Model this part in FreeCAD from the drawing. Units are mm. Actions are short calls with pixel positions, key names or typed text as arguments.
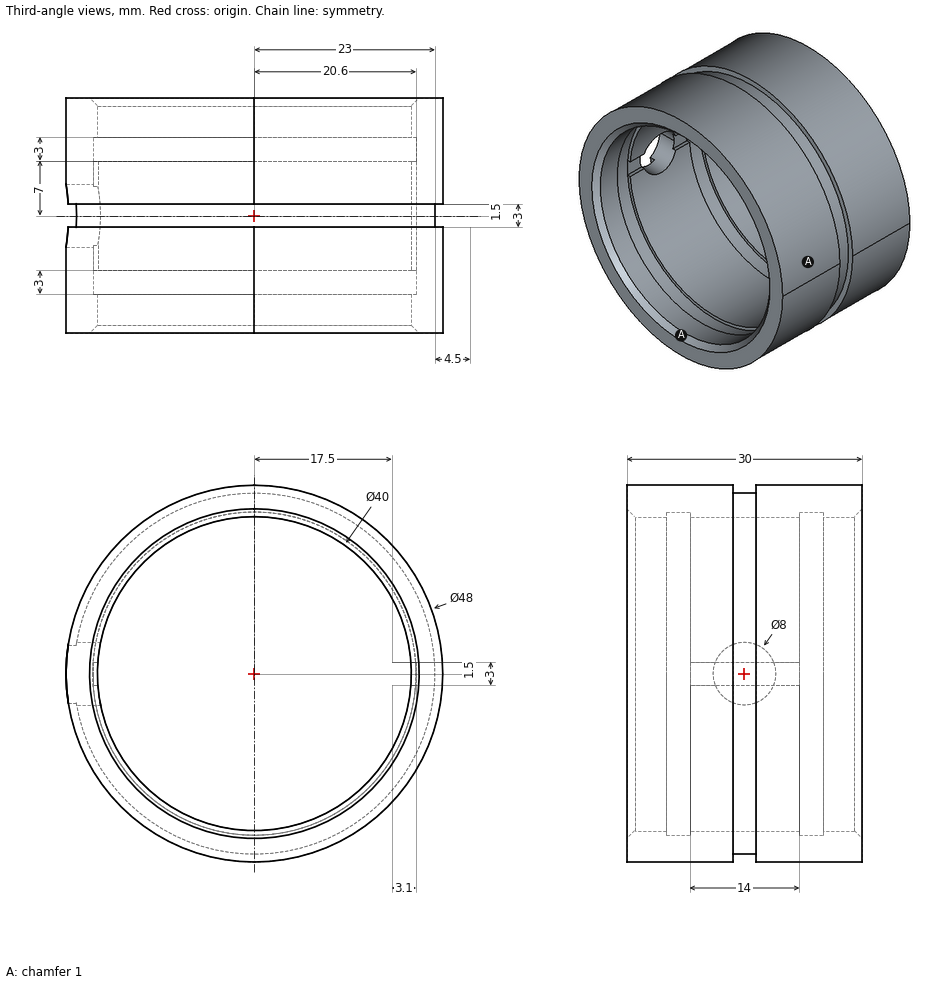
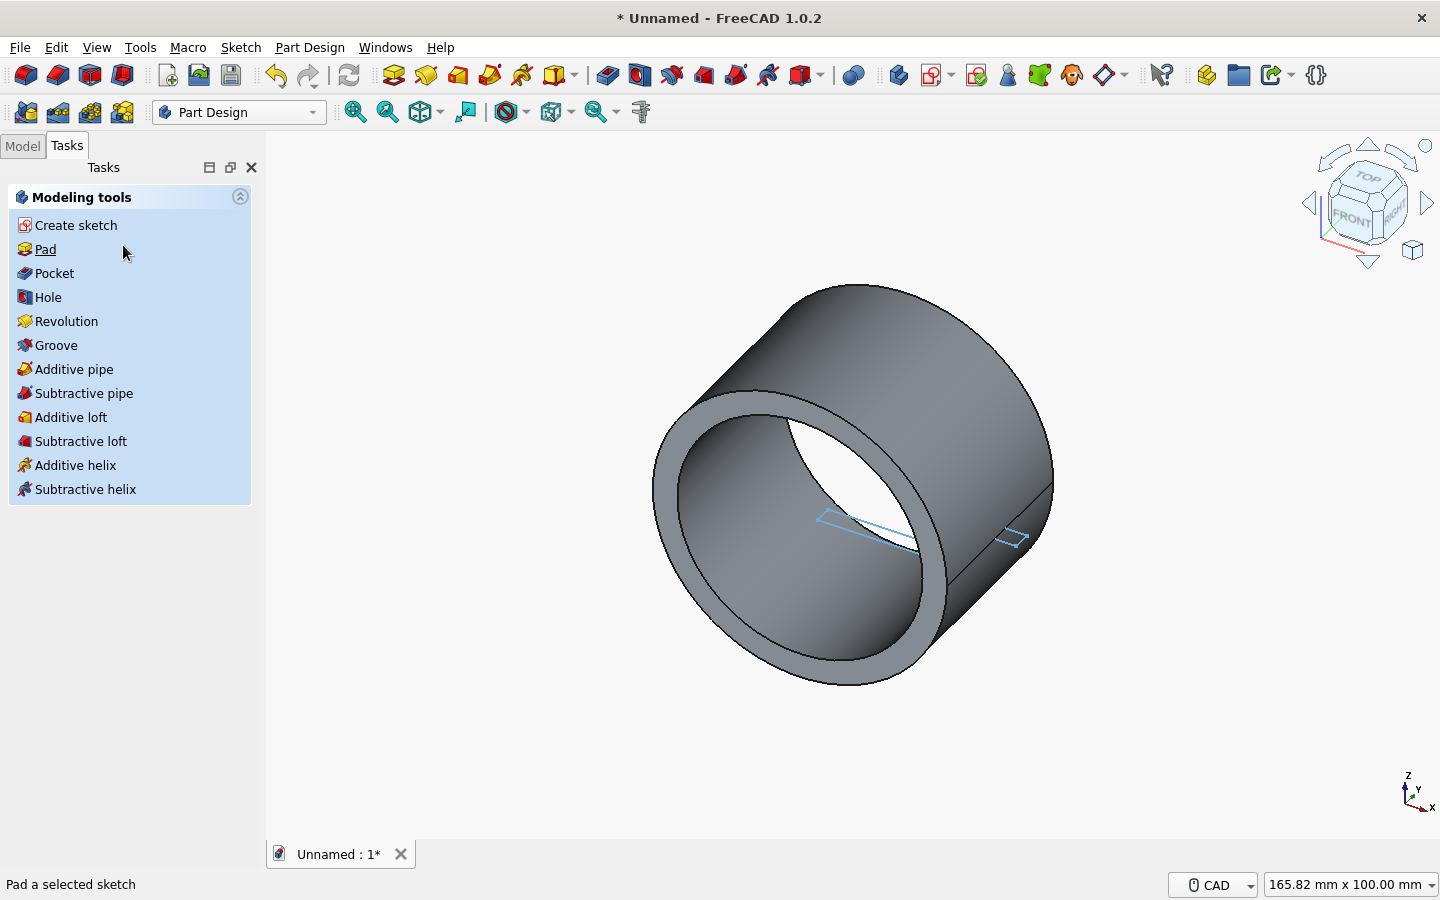
click(672, 76)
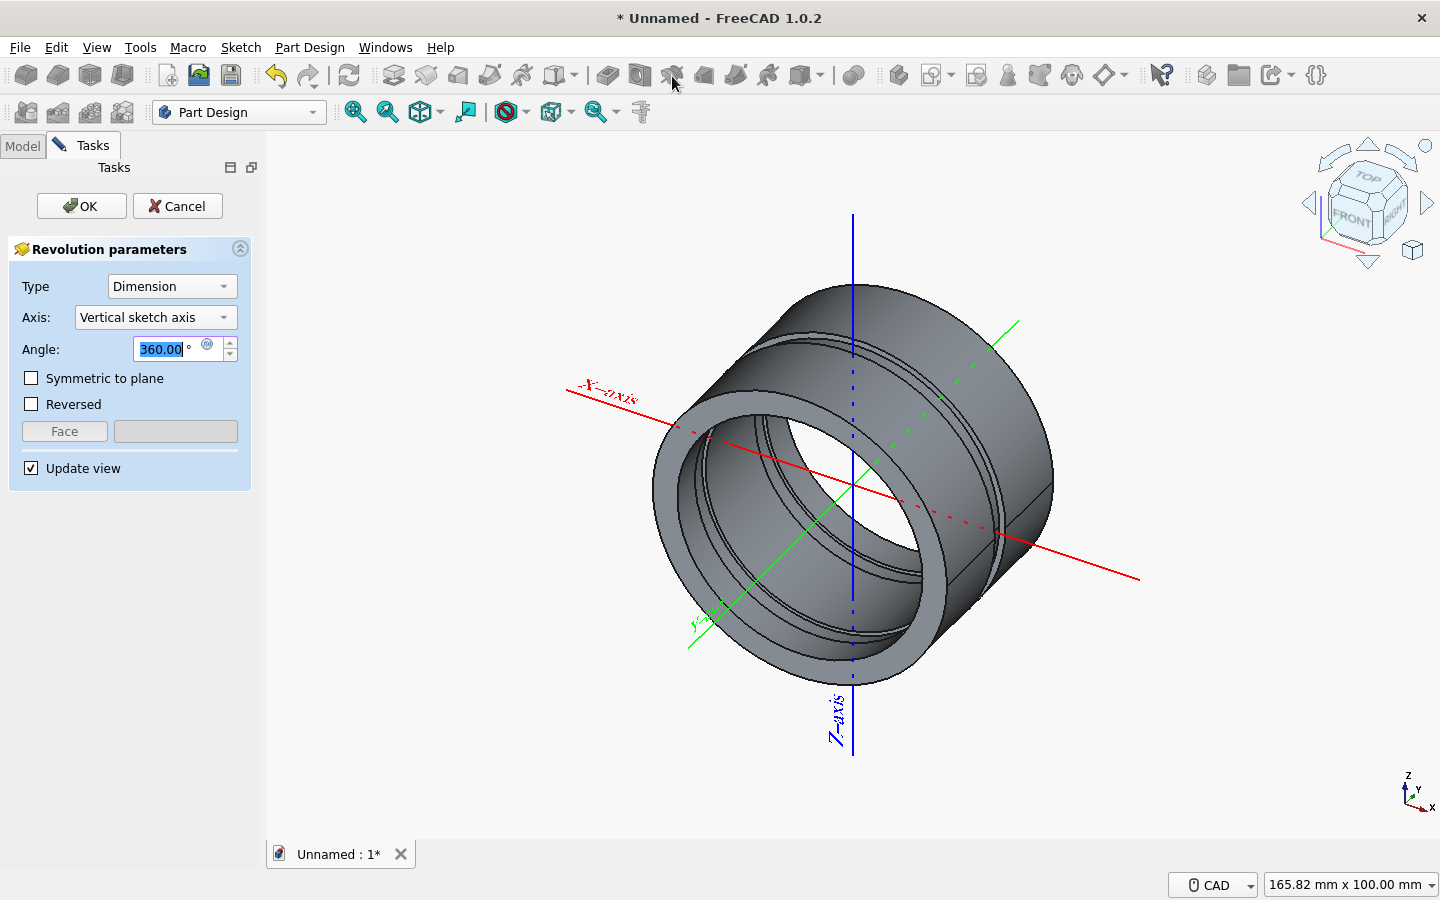
click(82, 206)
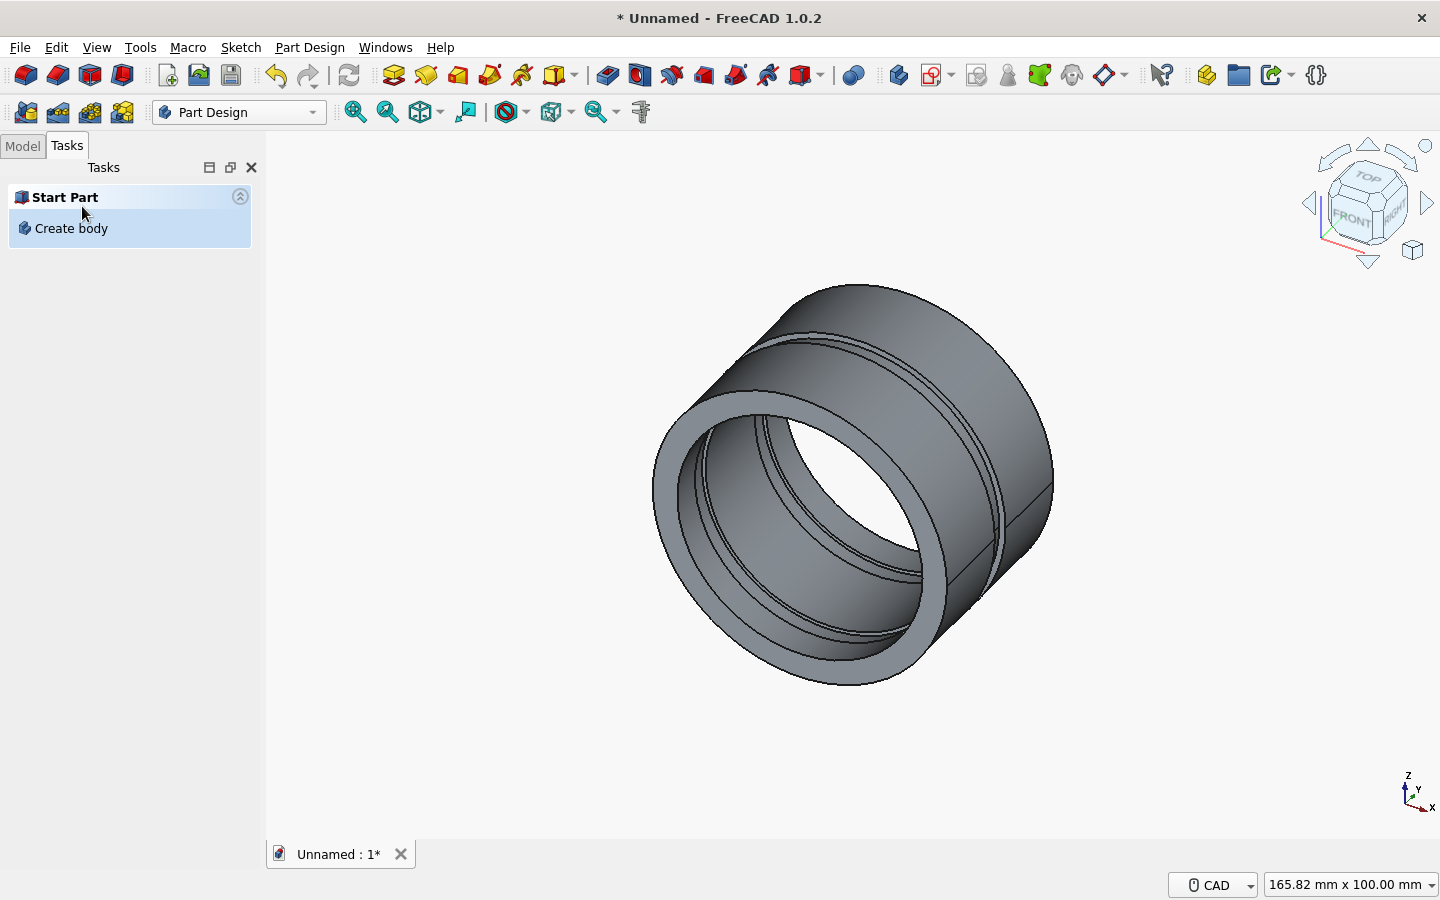
click(932, 76)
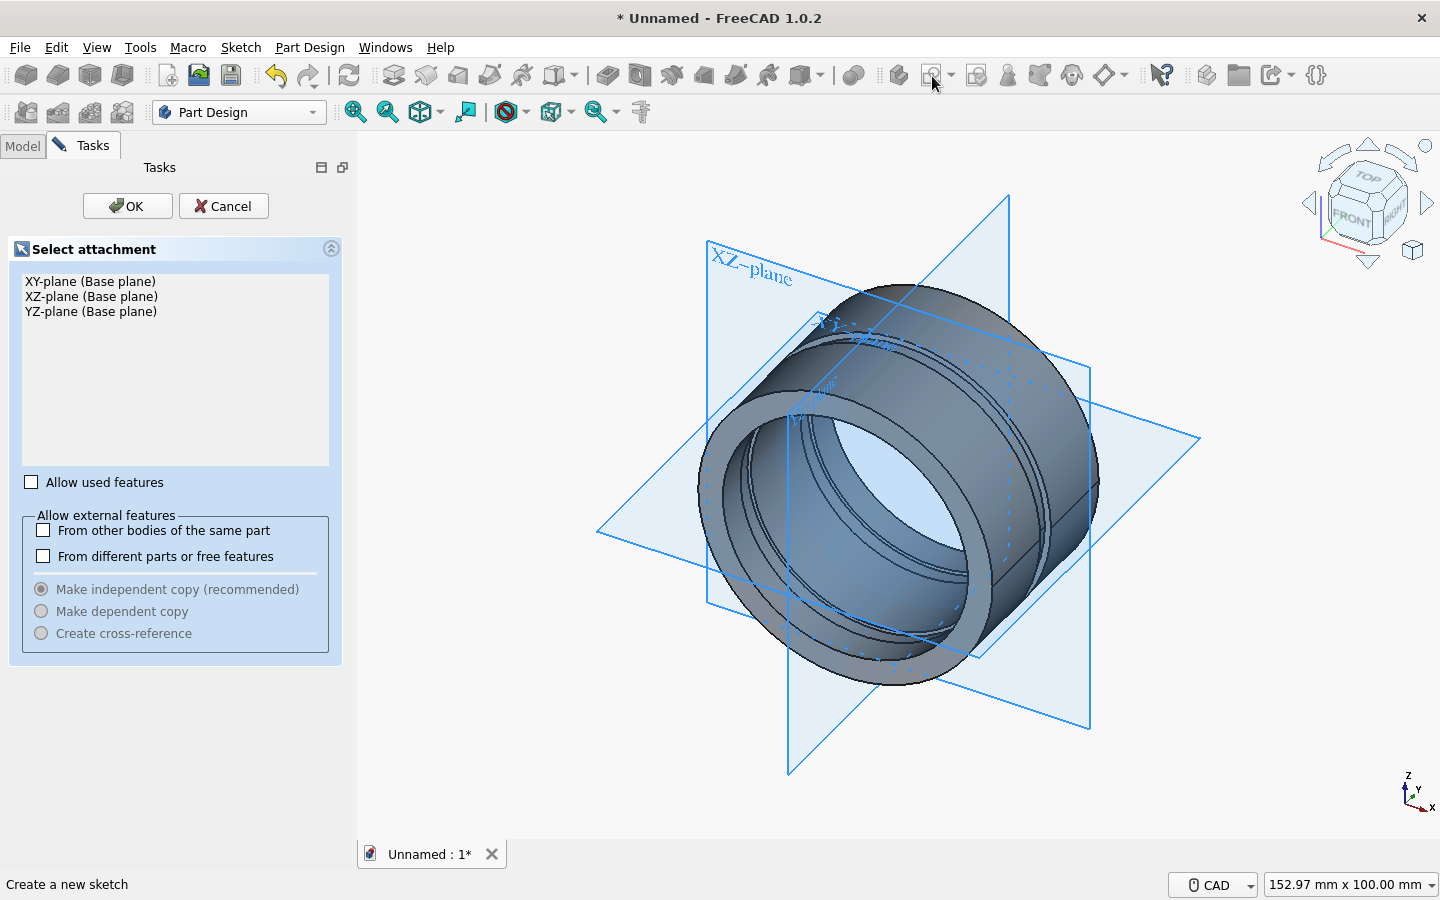
click(82, 296)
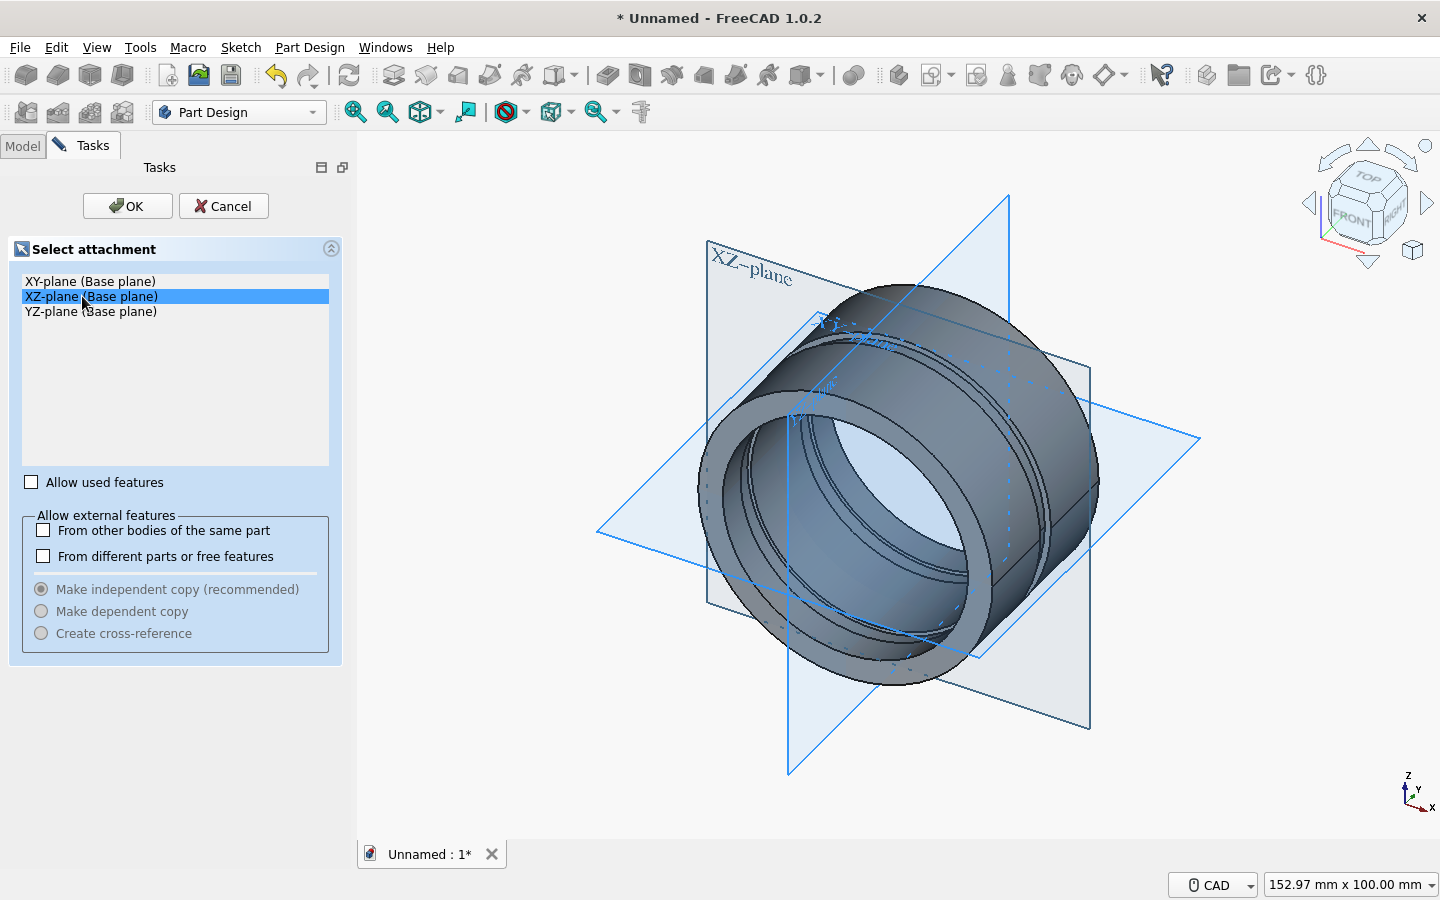
click(128, 206)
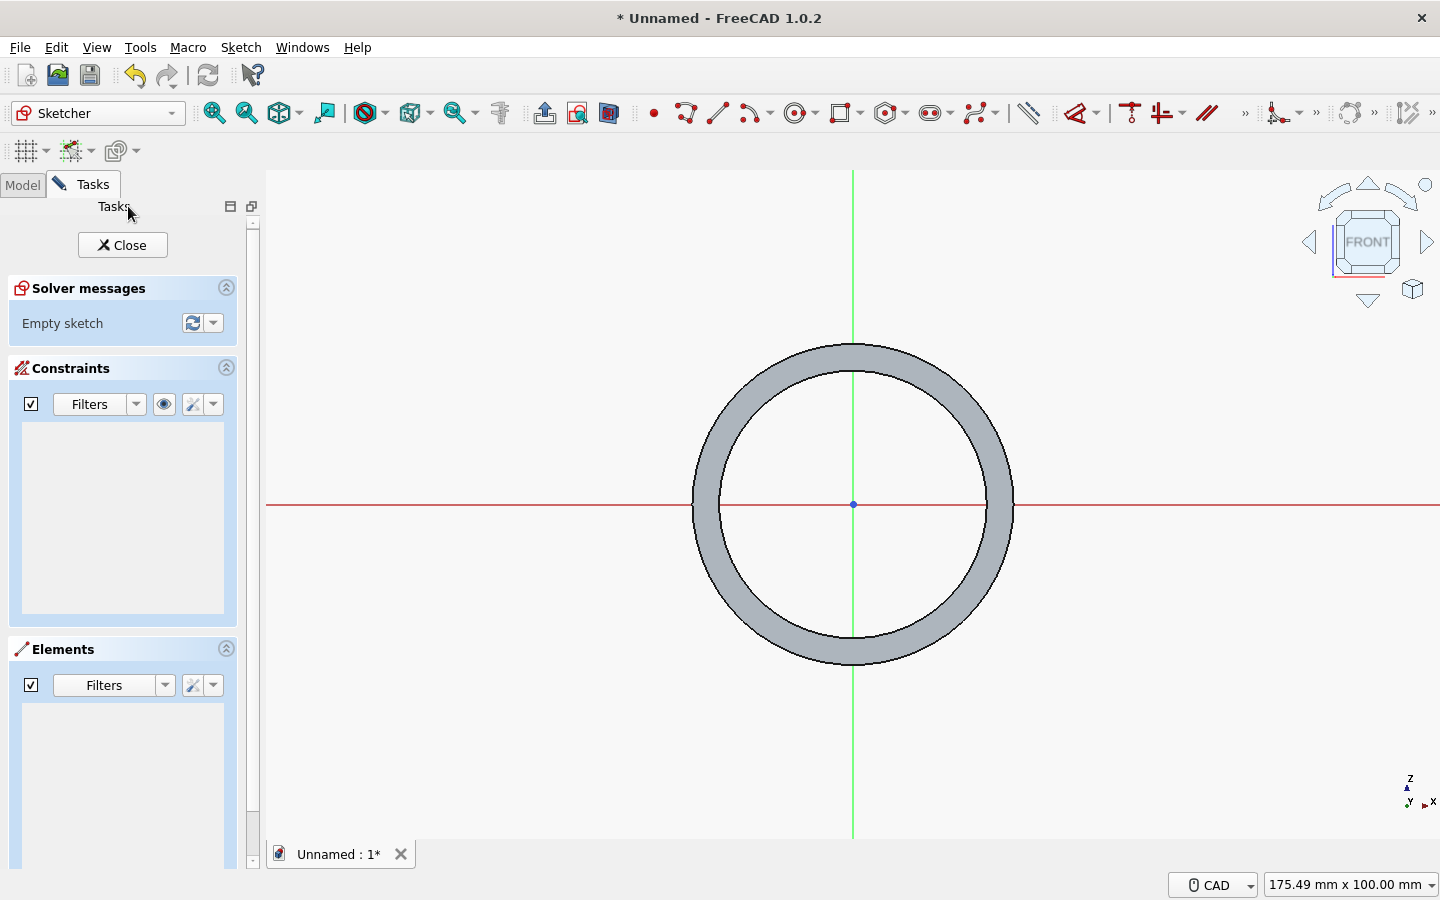
click(610, 114)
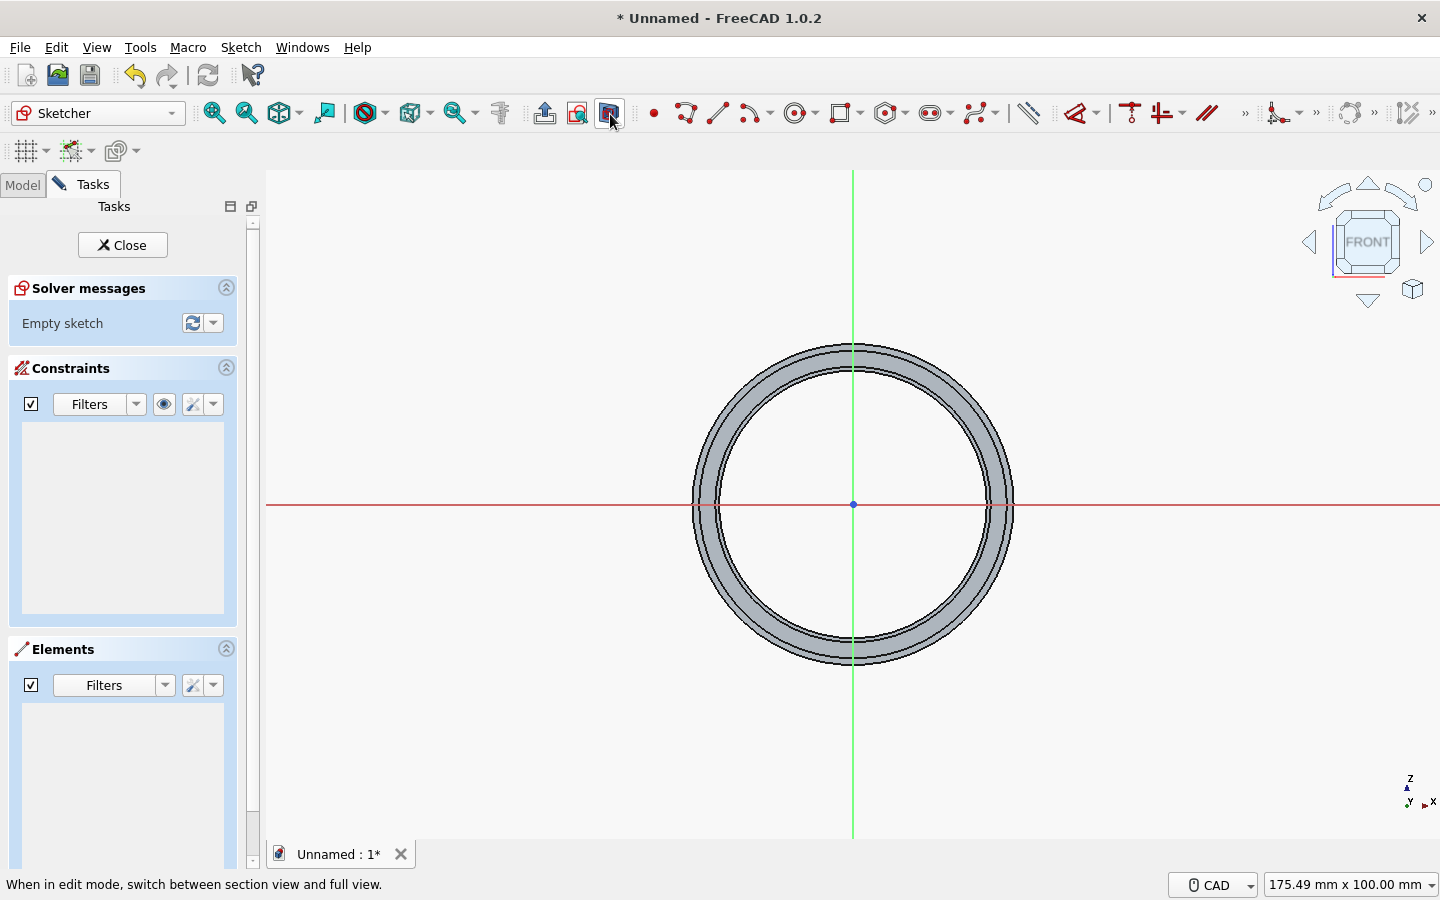
scroll(893, 504, up, 5)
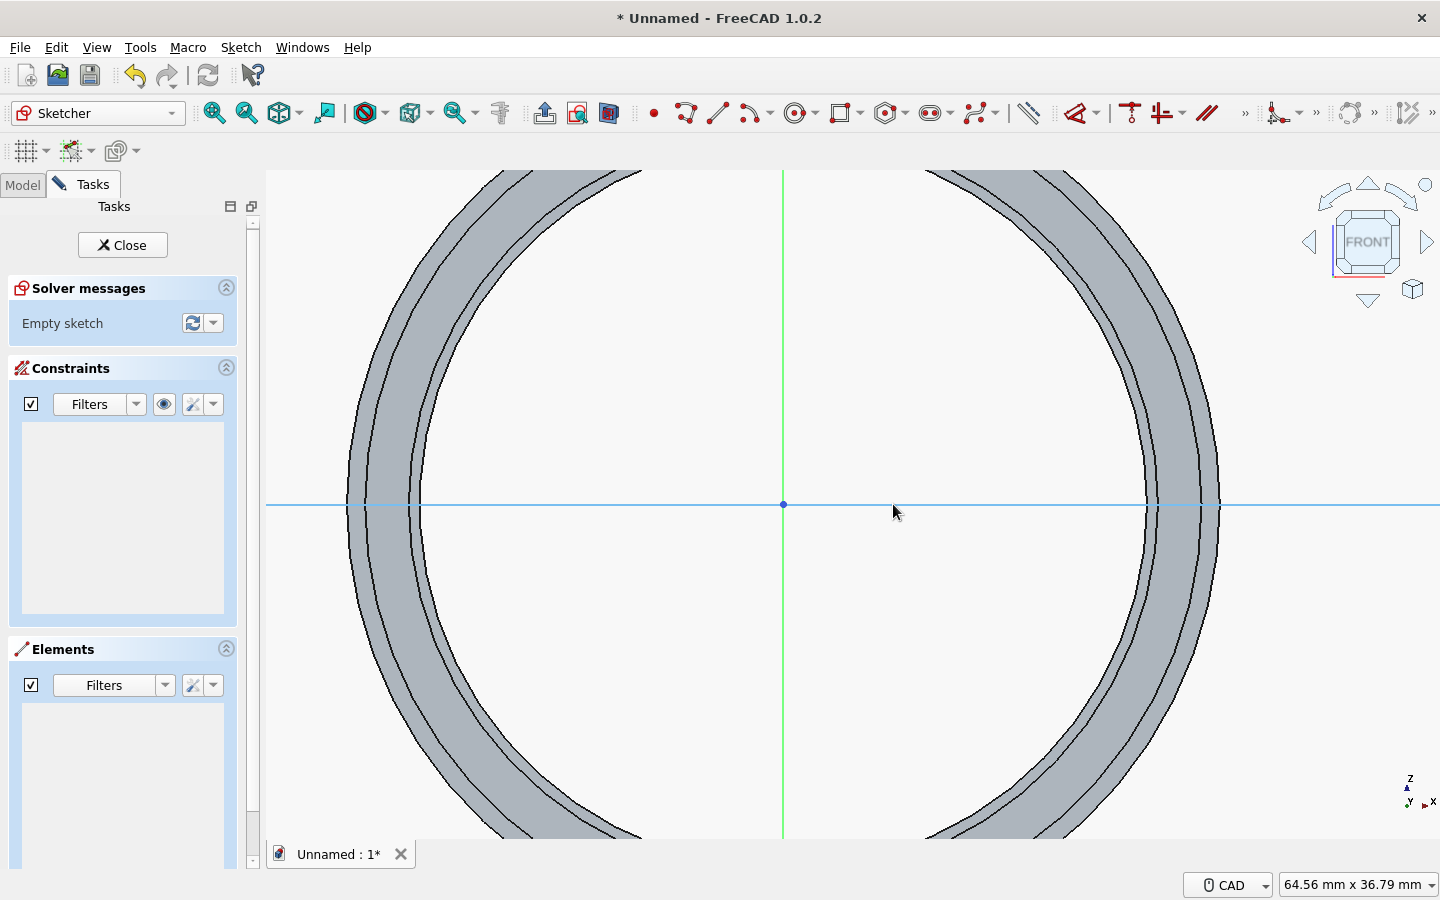
click(840, 114)